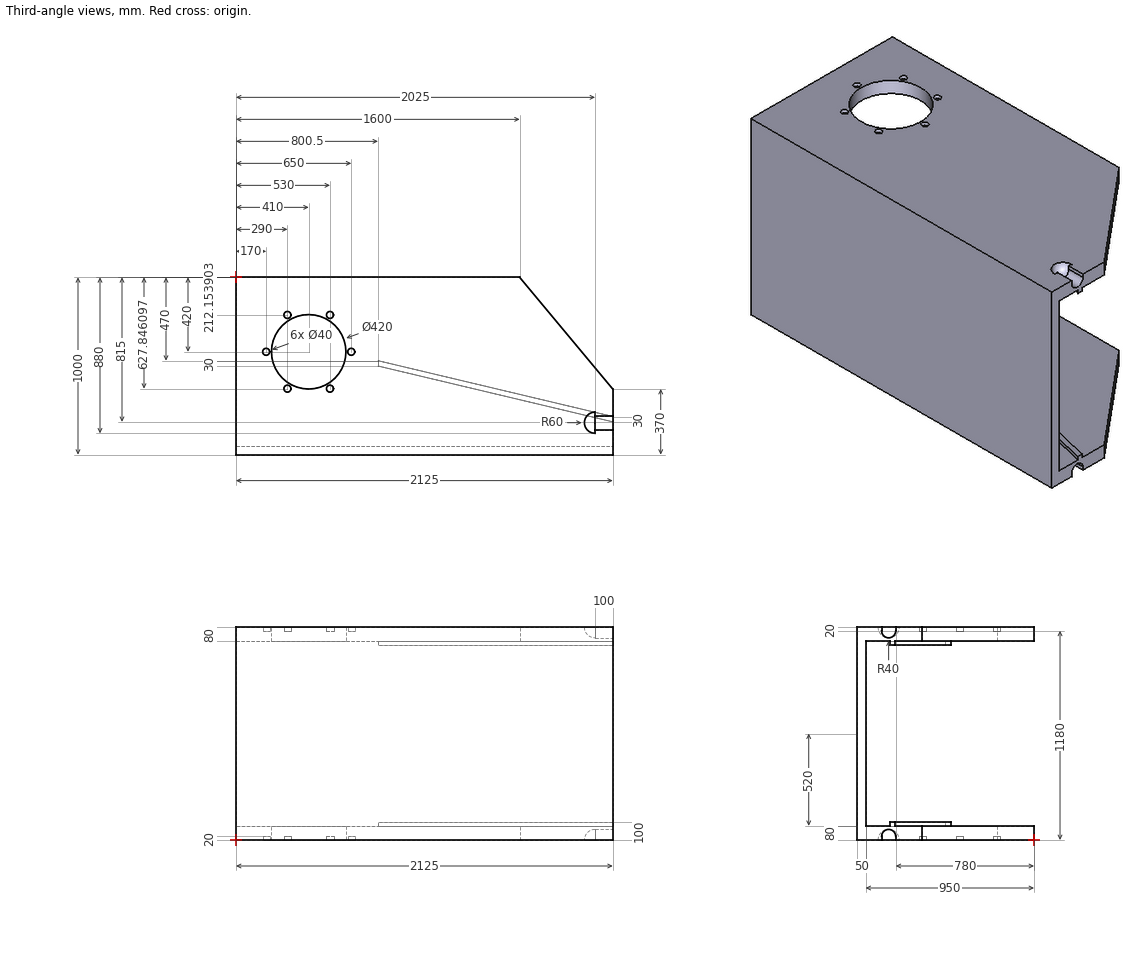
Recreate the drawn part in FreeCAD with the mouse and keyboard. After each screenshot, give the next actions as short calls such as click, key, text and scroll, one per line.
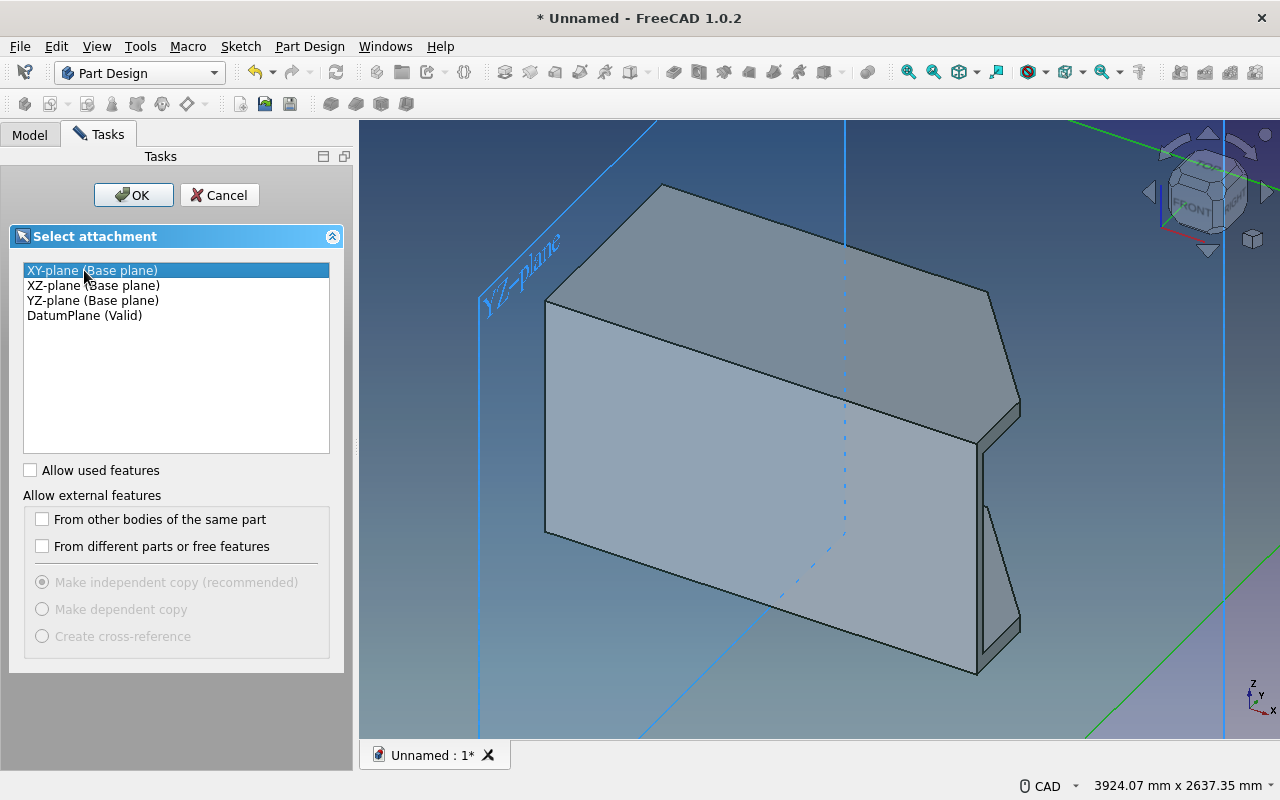
click(134, 195)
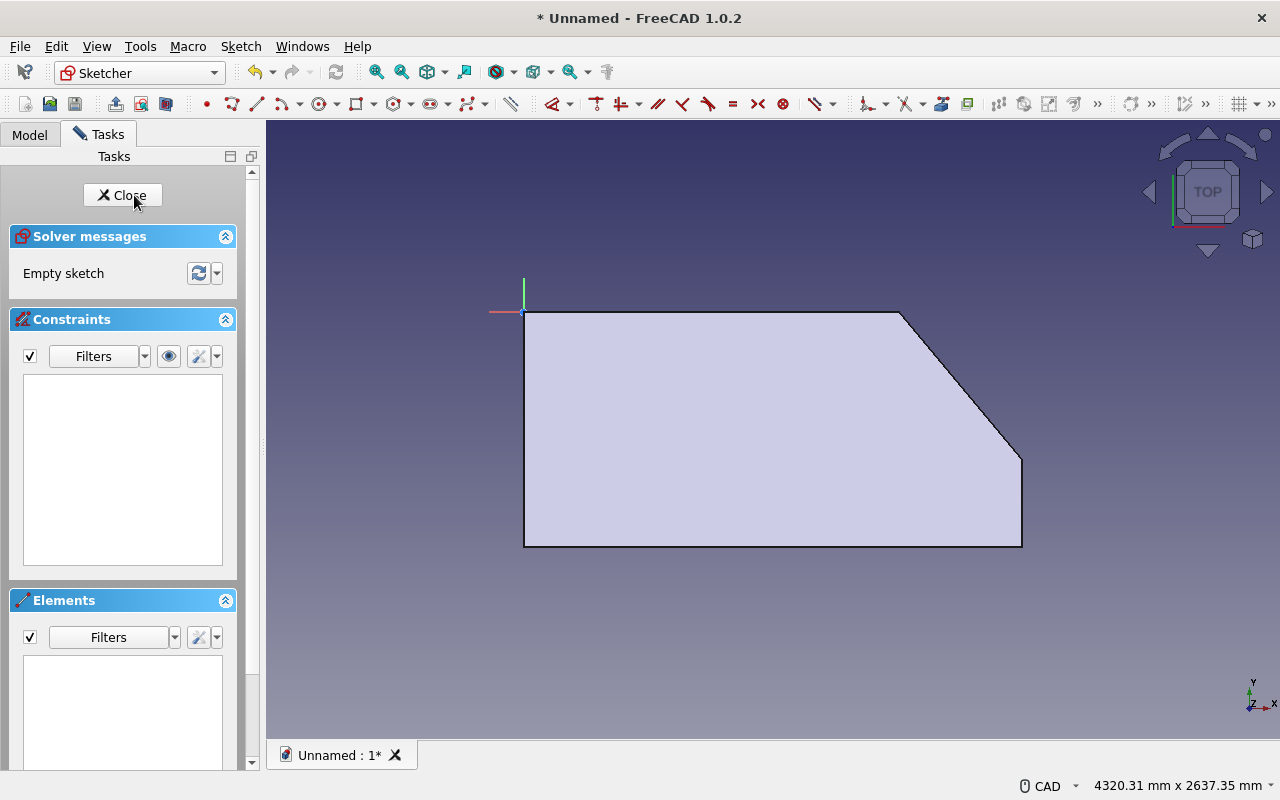
click(166, 104)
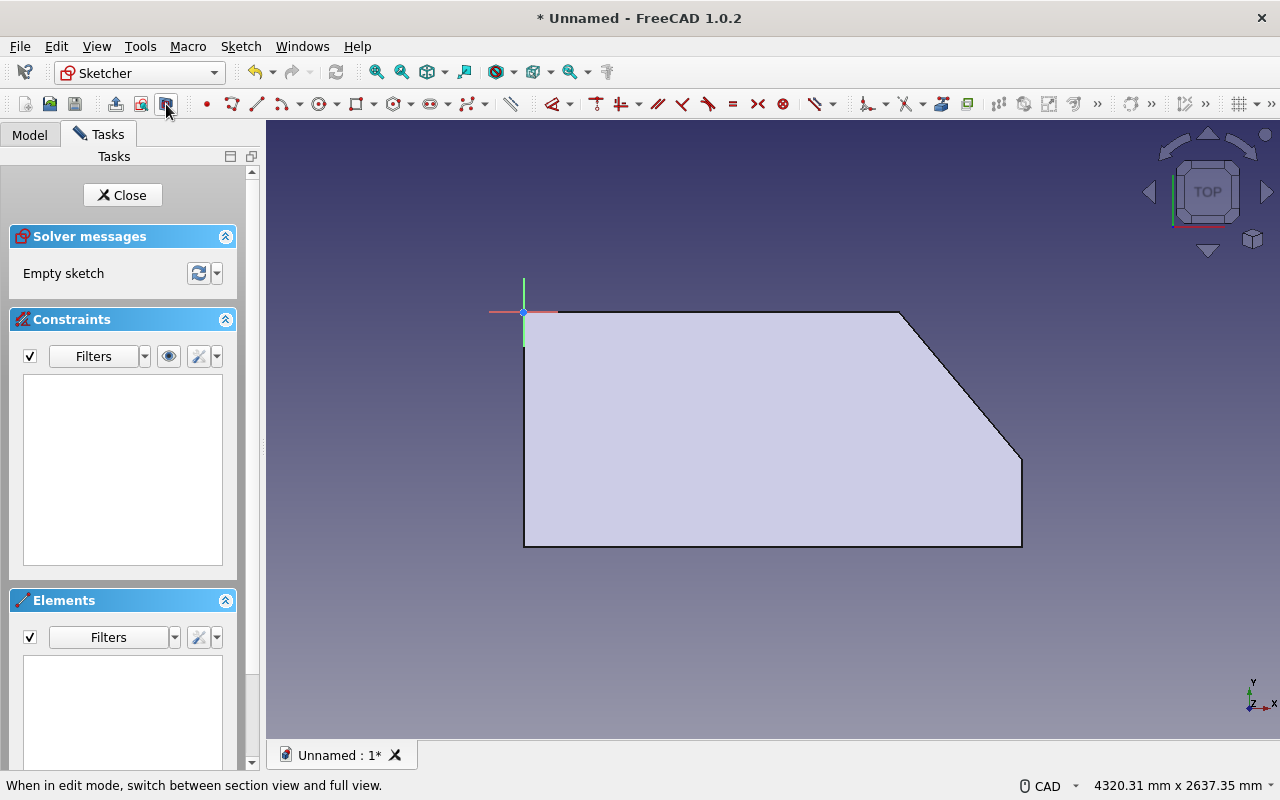
scroll(533, 361, up, 5)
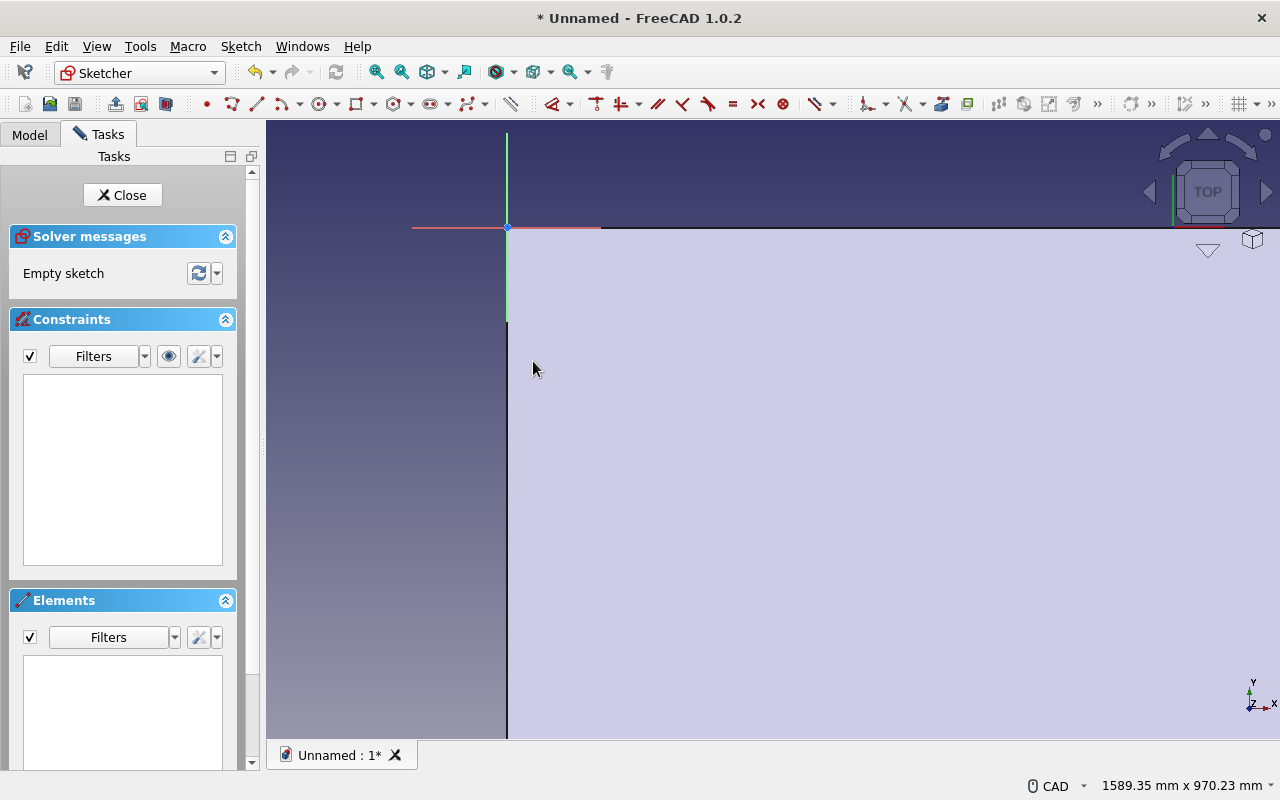
key(g)
key(c)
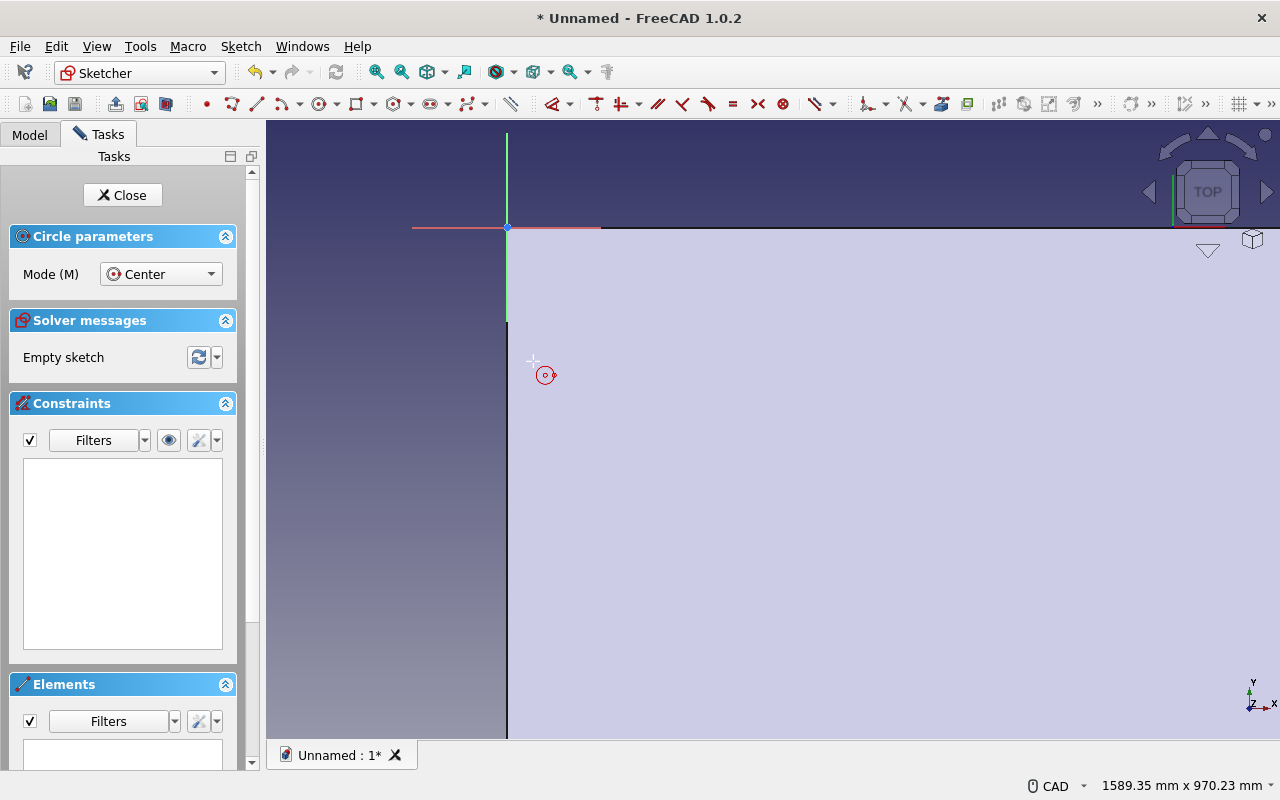
click(769, 495)
click(863, 401)
key(Escape)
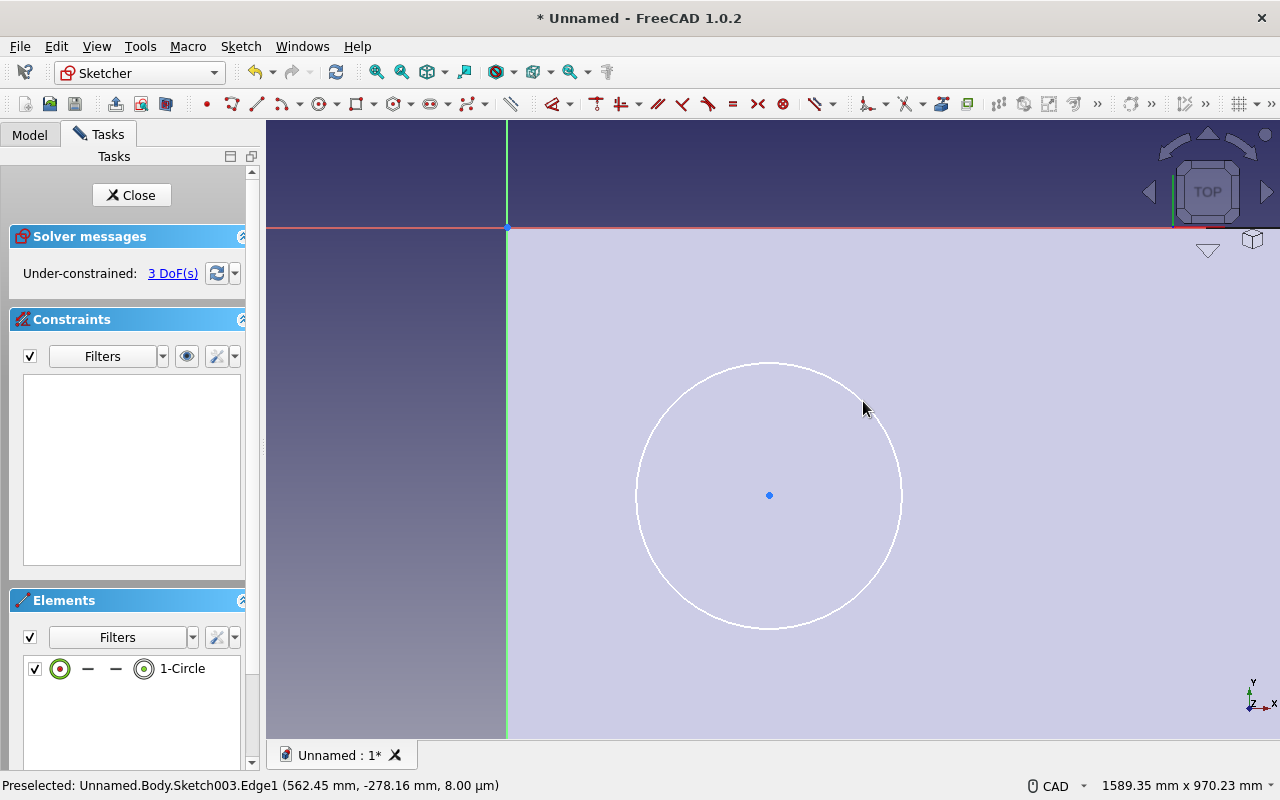
key(d)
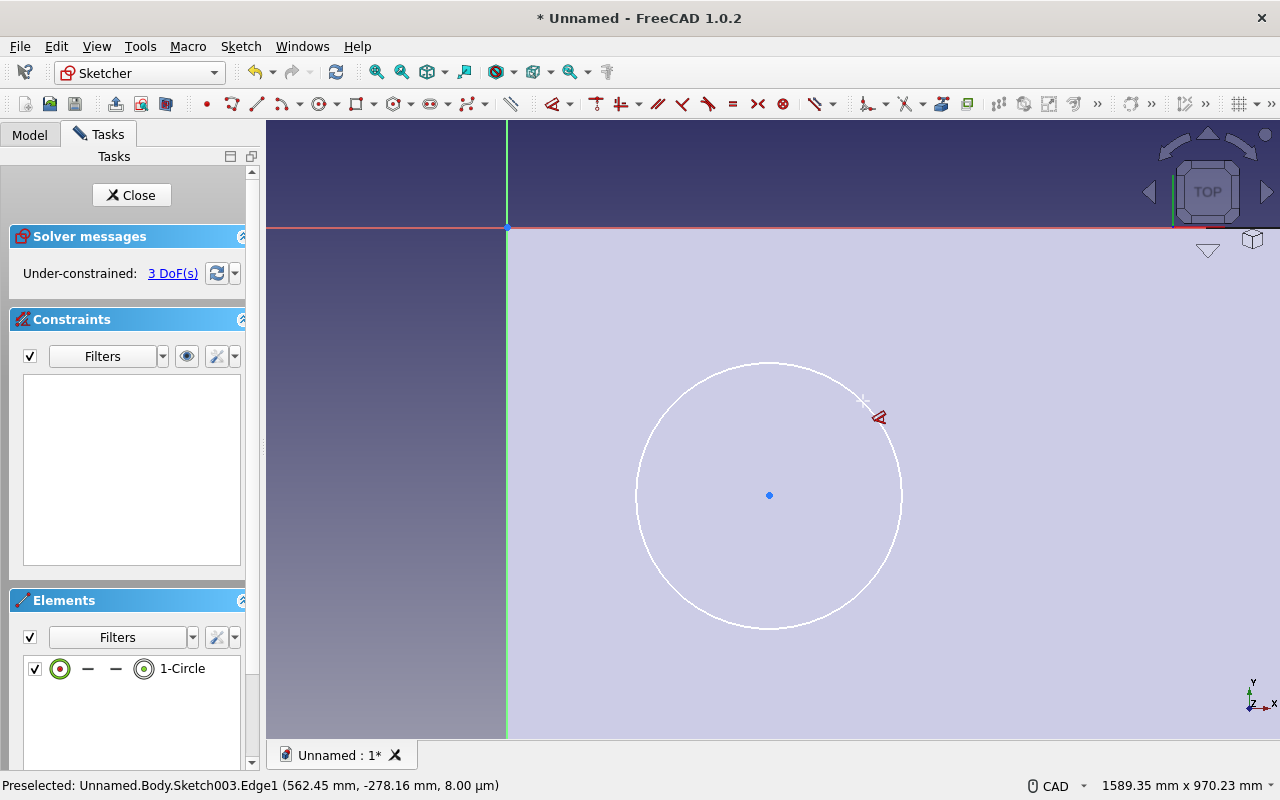
click(863, 402)
click(886, 379)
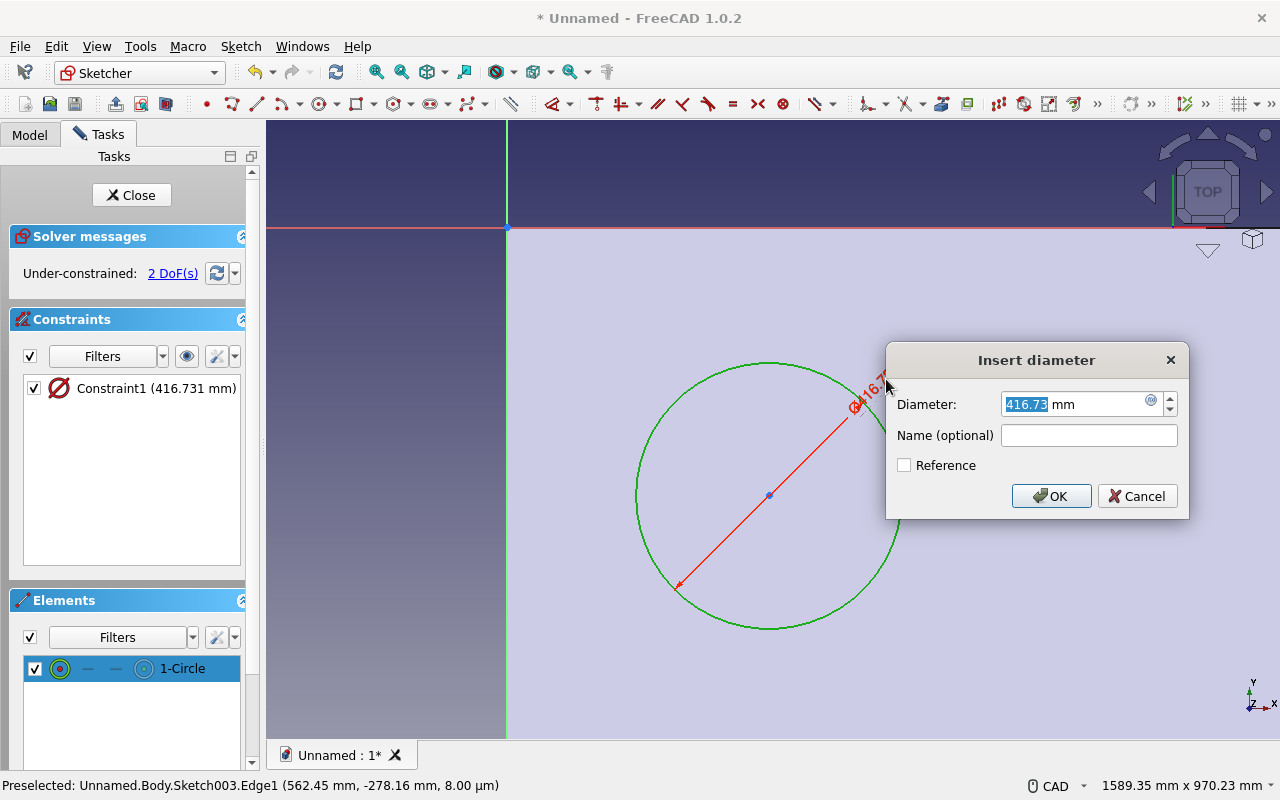
text(420)
key(Return)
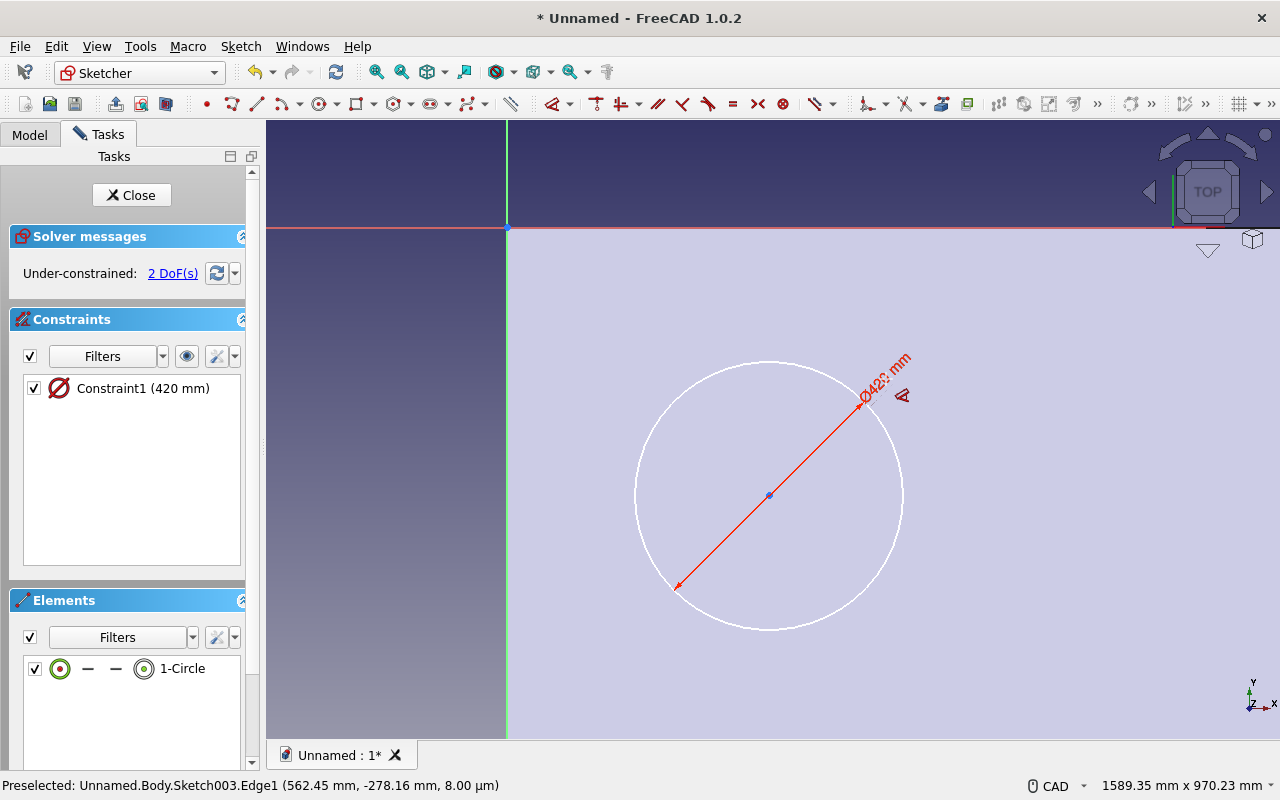
click(769, 496)
click(638, 194)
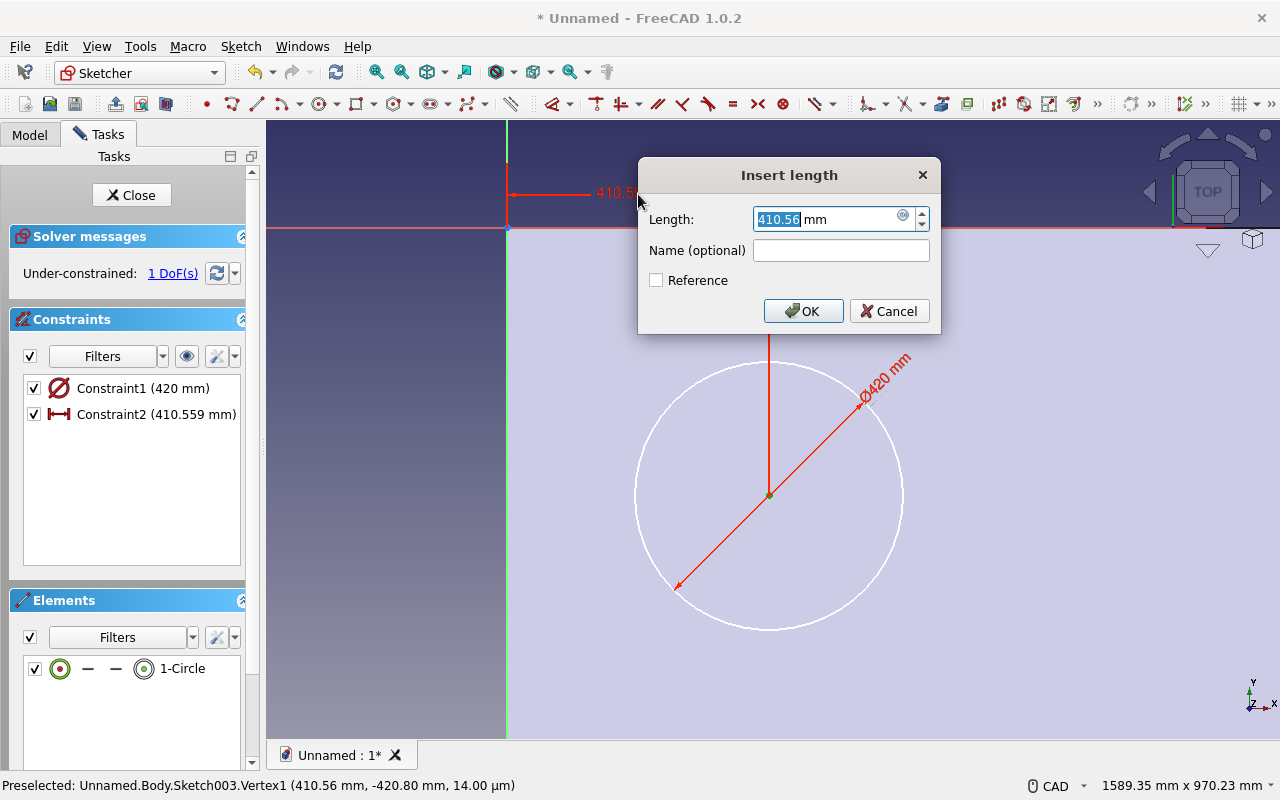
text(410)
key(Return)